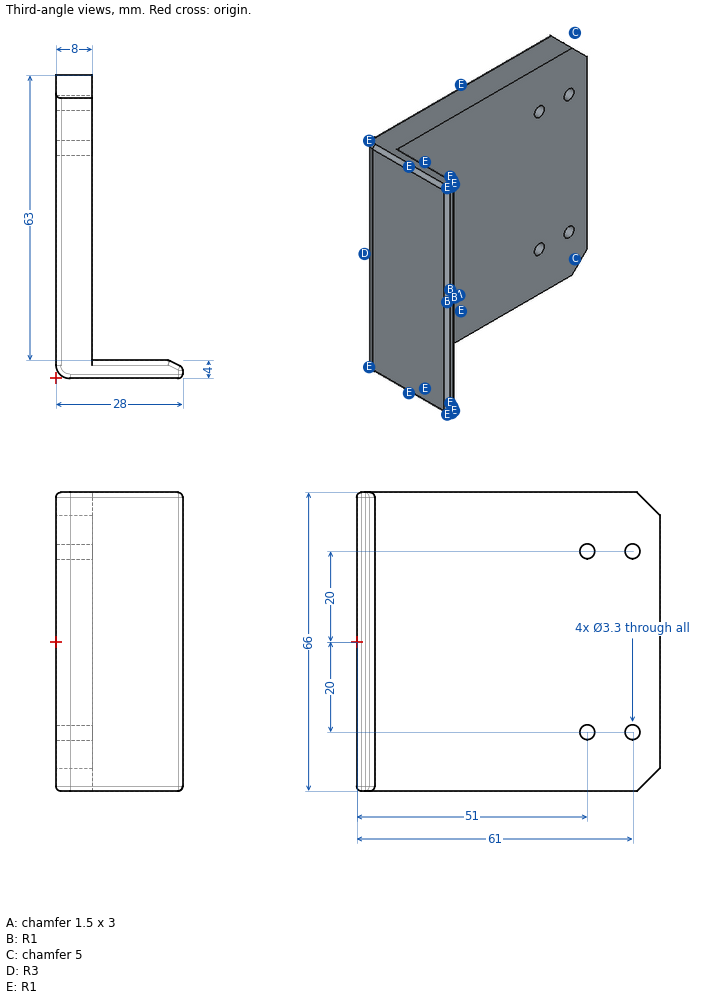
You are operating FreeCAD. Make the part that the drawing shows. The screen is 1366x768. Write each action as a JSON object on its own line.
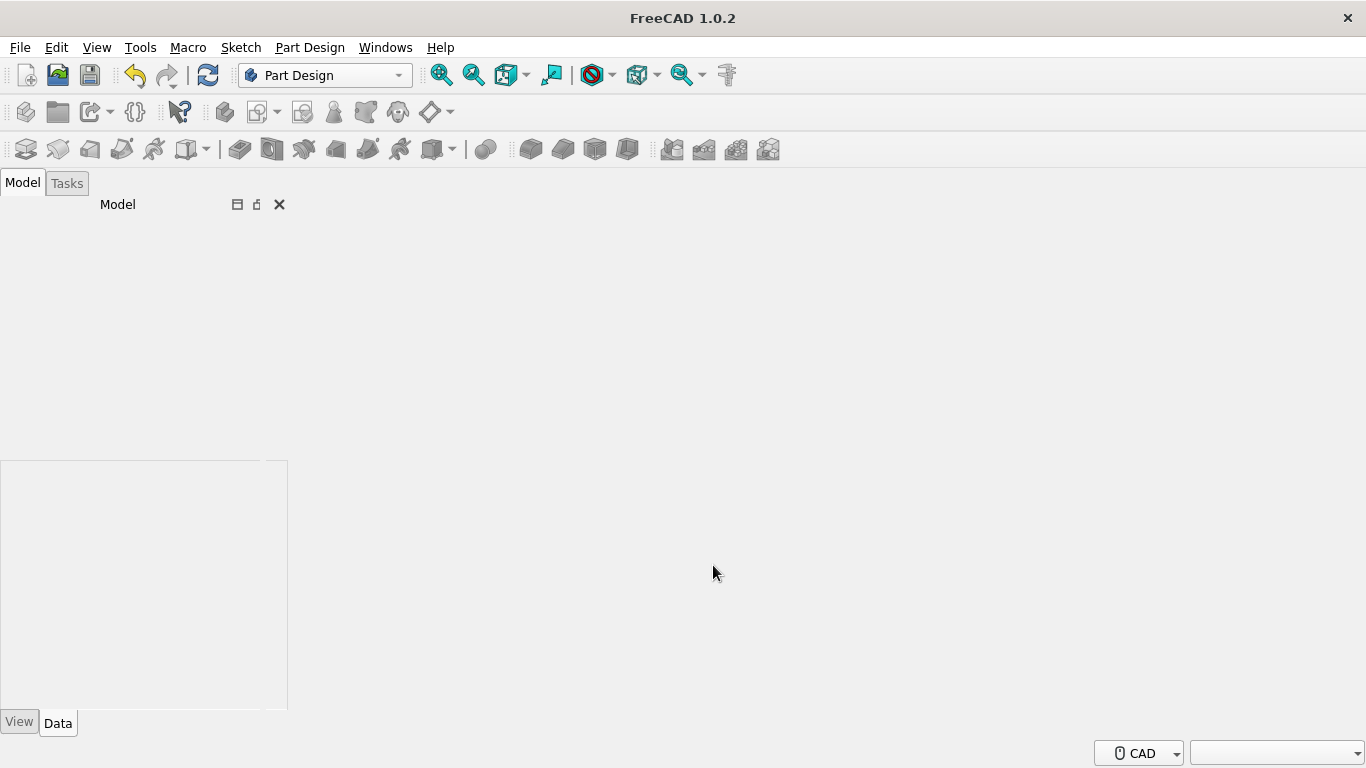
{"action": "key", "text": "ctrl+n"}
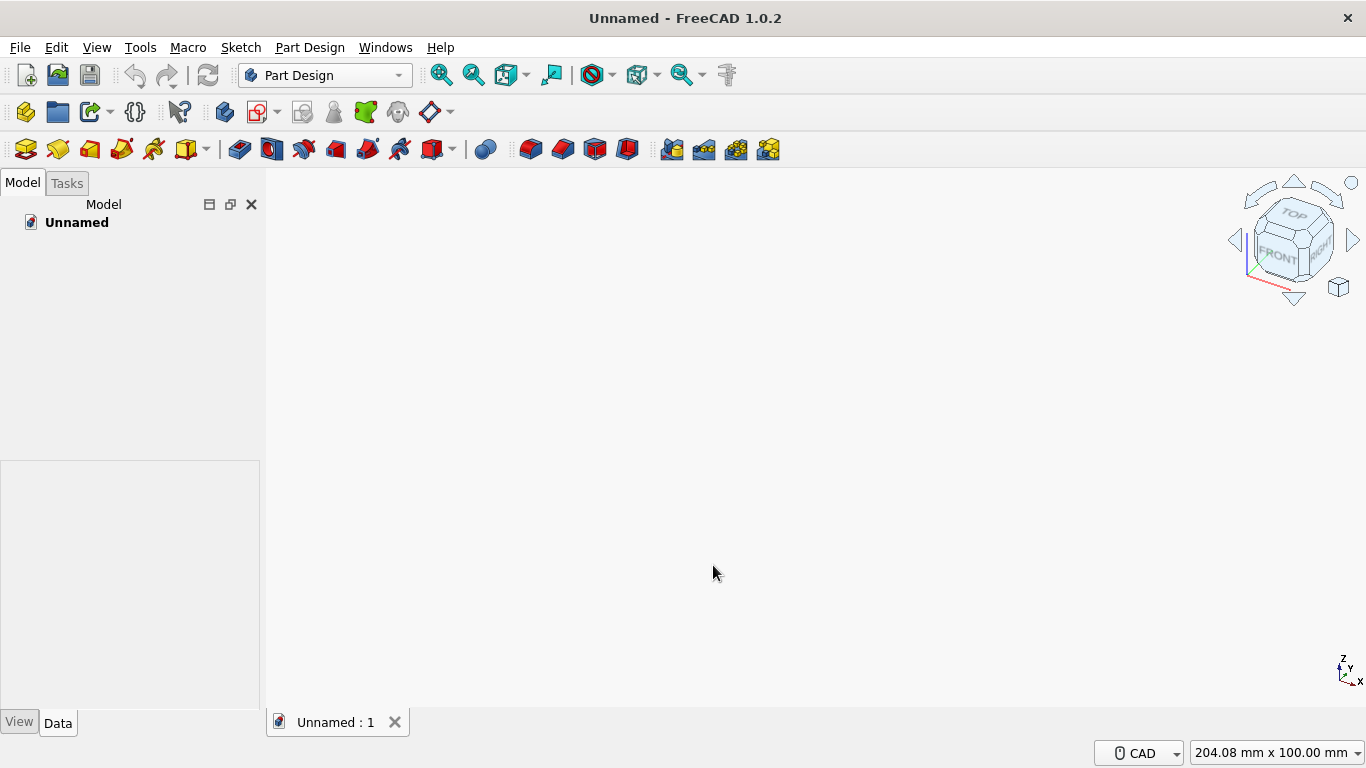
{"action": "left_click", "coordinate": [258, 112]}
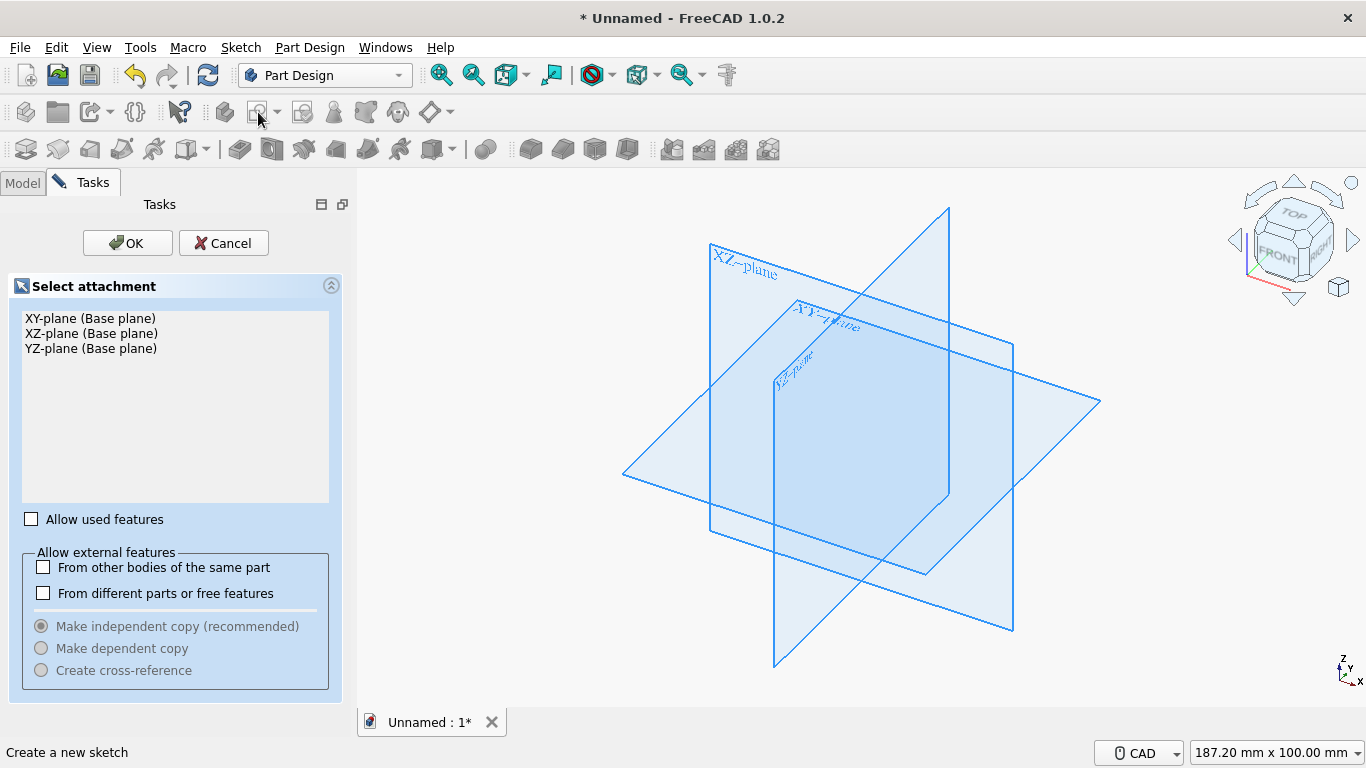
{"action": "left_click", "coordinate": [82, 318]}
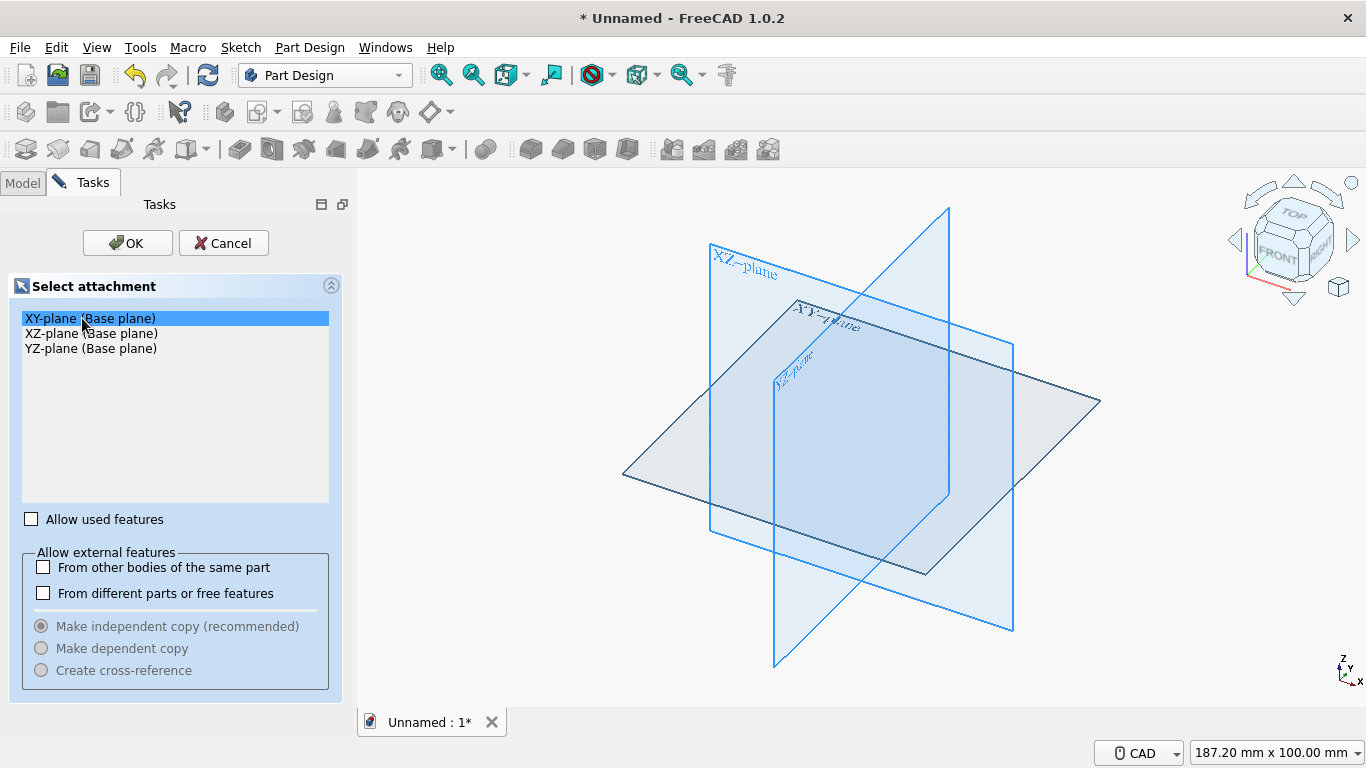
{"action": "left_click", "coordinate": [128, 243]}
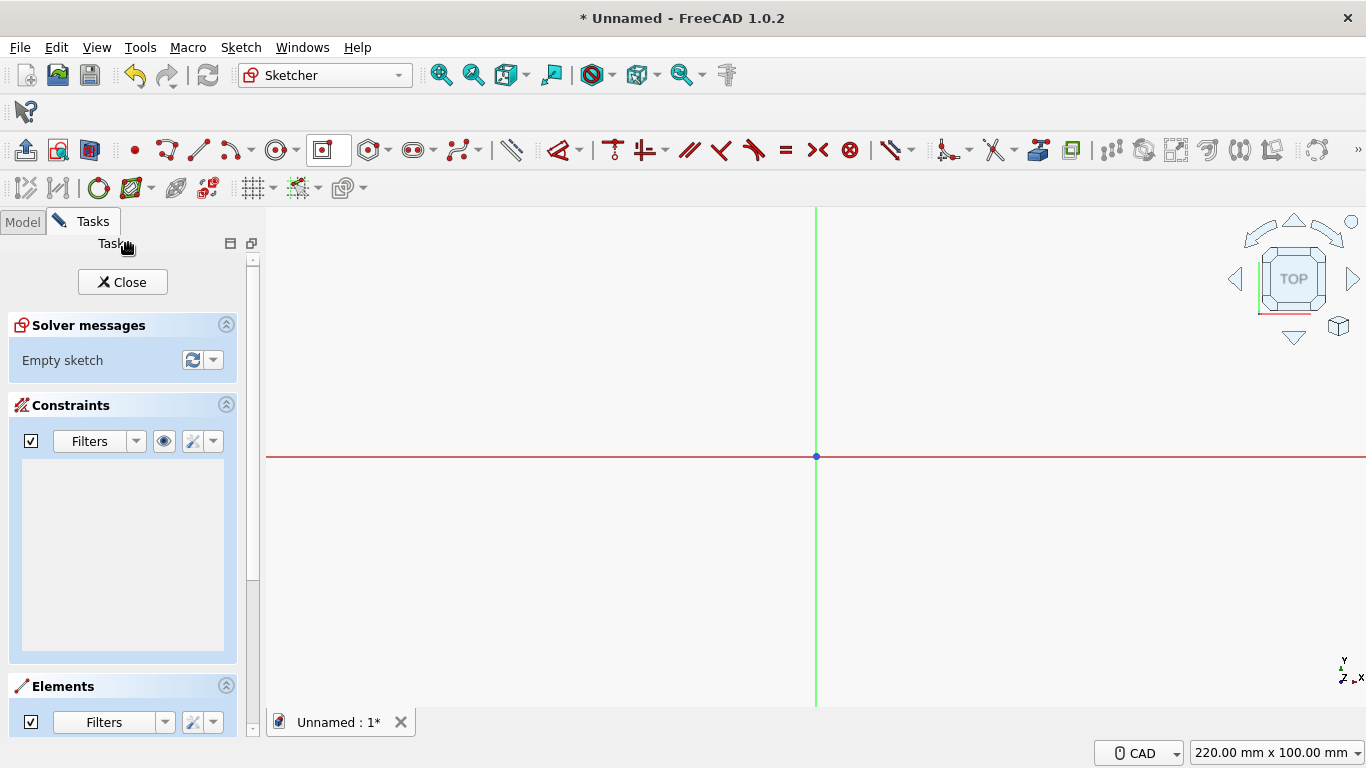
{"action": "scroll", "coordinate": [466, 679], "scroll_direction": "down", "scroll_amount": 2}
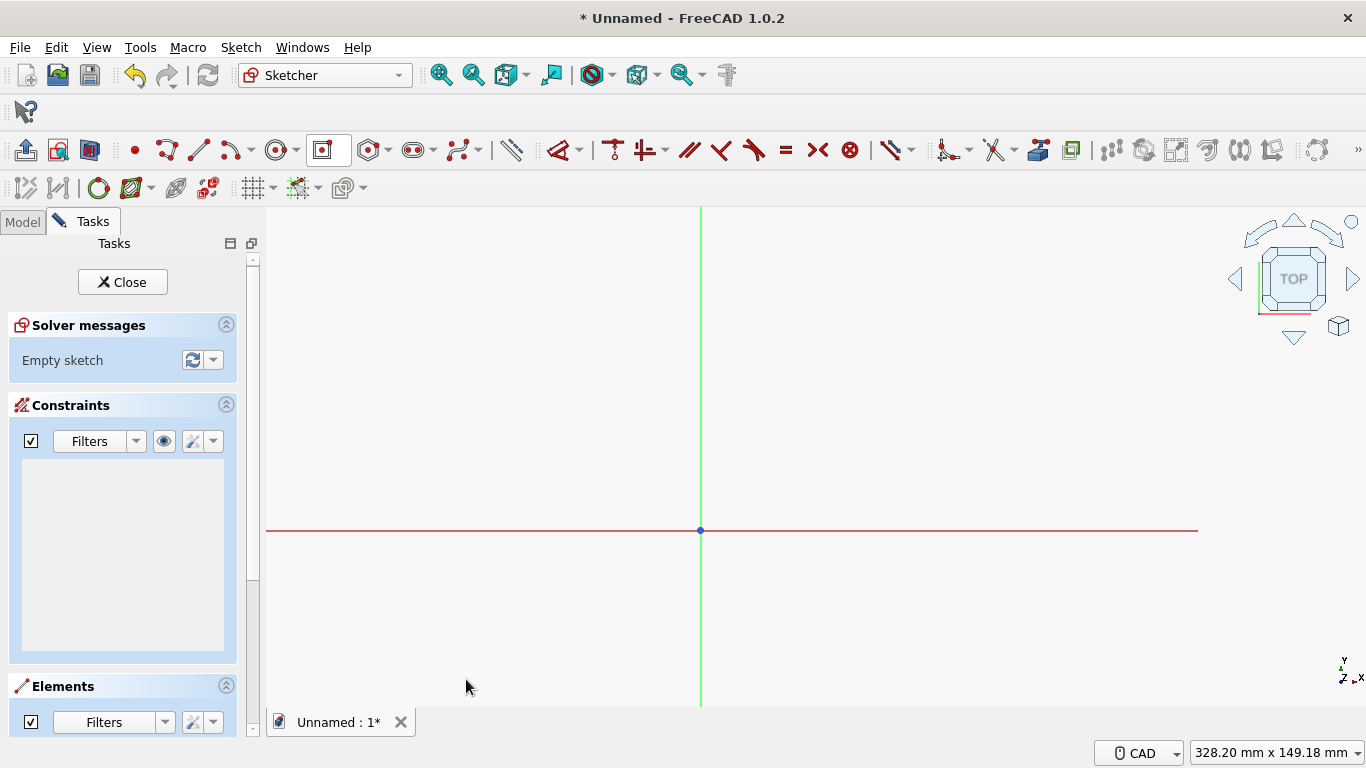
{"action": "scroll", "coordinate": [748, 339], "scroll_direction": "up", "scroll_amount": 2}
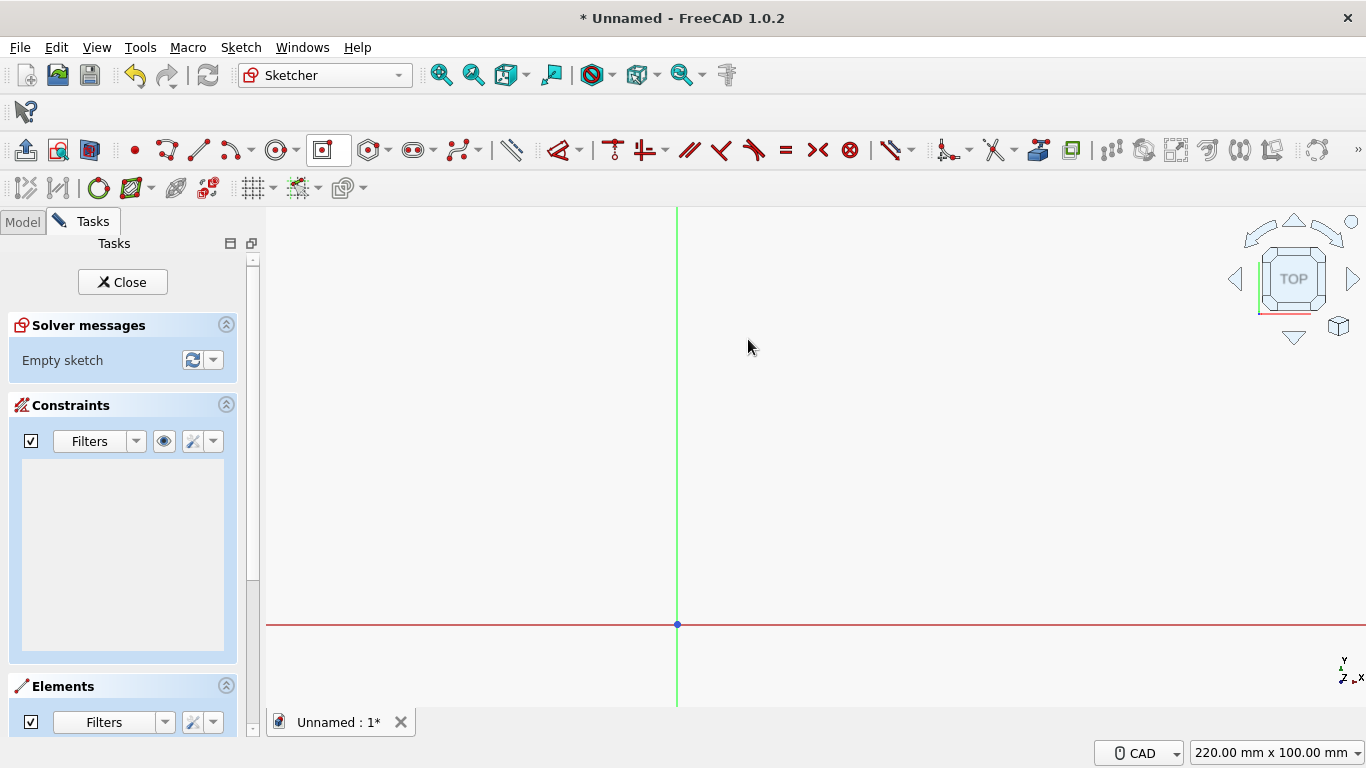
{"action": "left_click", "coordinate": [168, 150]}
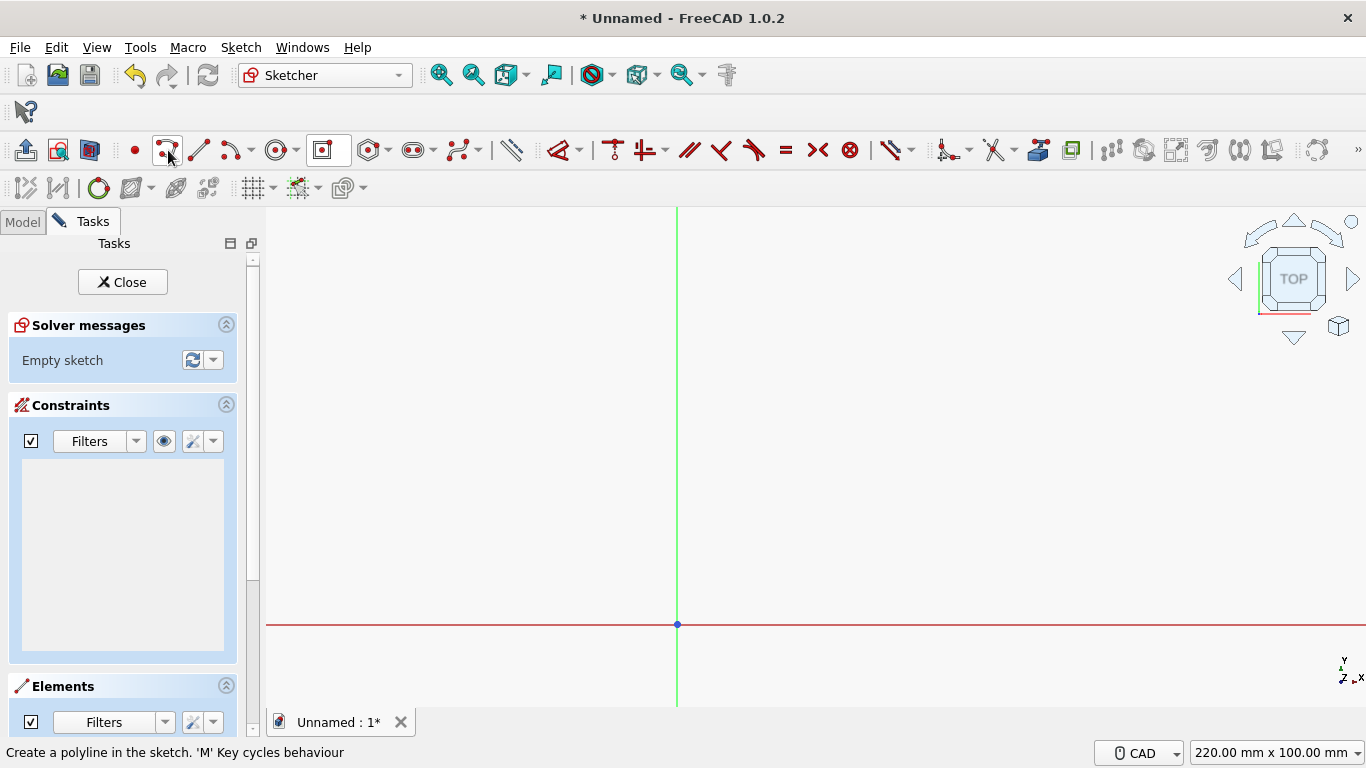
{"action": "left_click", "coordinate": [677, 625]}
{"action": "left_click", "coordinate": [817, 616]}
{"action": "left_click", "coordinate": [817, 605]}
{"action": "left_click", "coordinate": [717, 605]}
{"action": "left_click", "coordinate": [717, 290]}
{"action": "left_click", "coordinate": [686, 290]}
{"action": "left_click", "coordinate": [677, 625]}
{"action": "key", "text": "Escape"}
{"action": "key", "text": "Escape"}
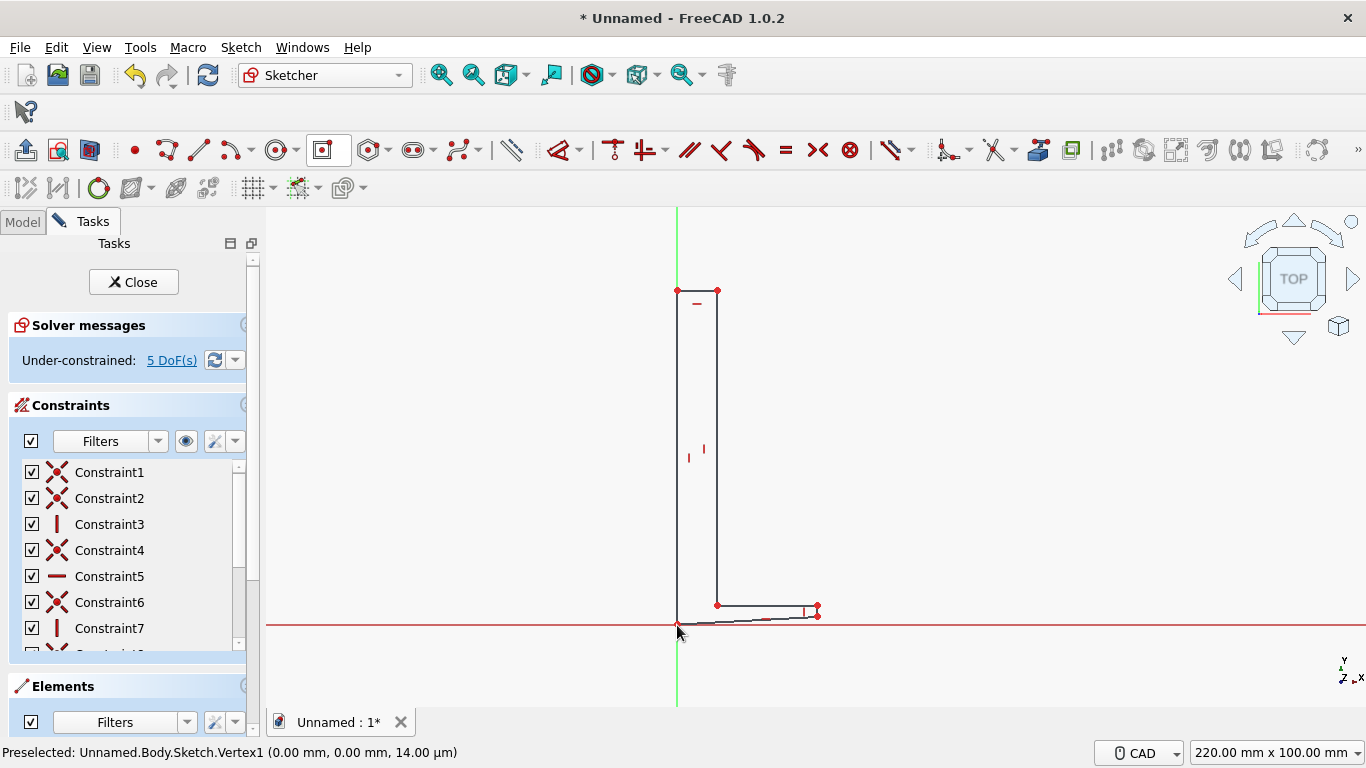
{"action": "left_click", "coordinate": [719, 622]}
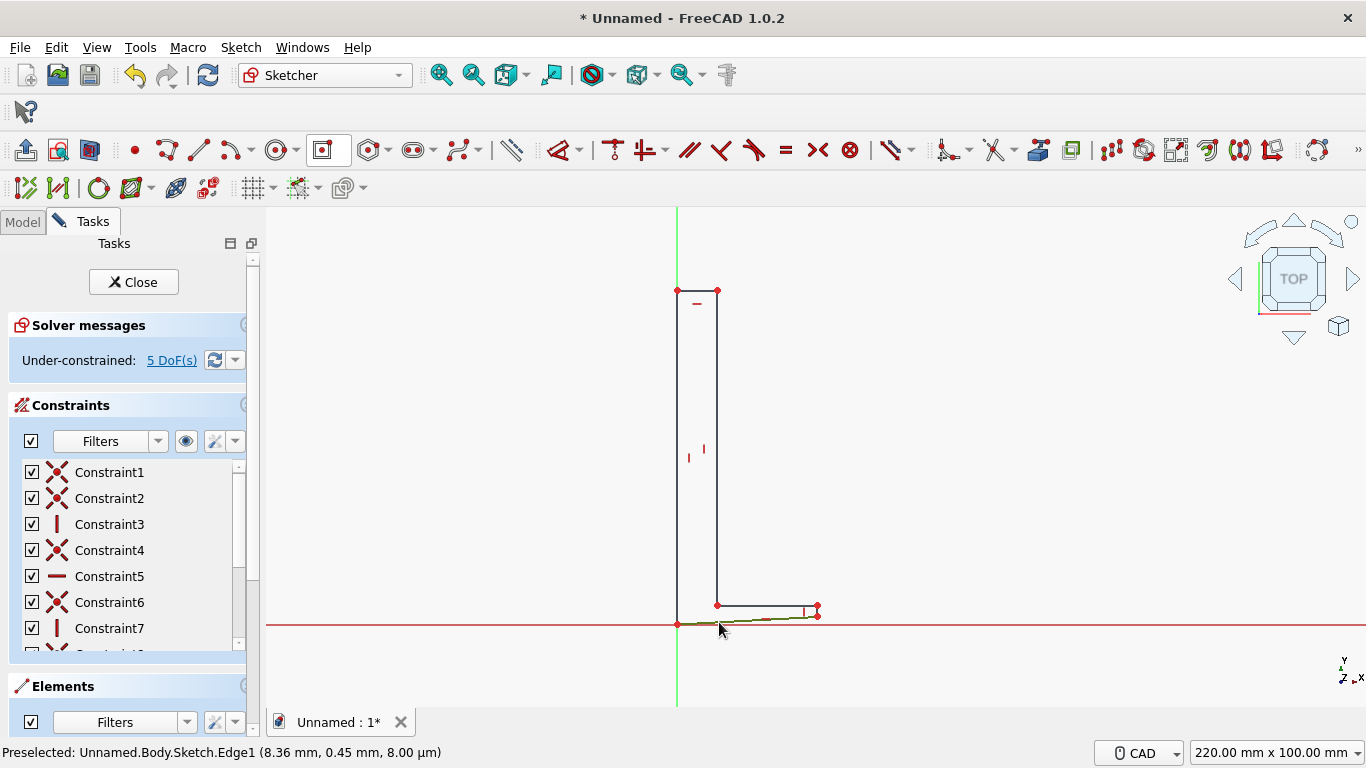
{"action": "left_click", "coordinate": [668, 150]}